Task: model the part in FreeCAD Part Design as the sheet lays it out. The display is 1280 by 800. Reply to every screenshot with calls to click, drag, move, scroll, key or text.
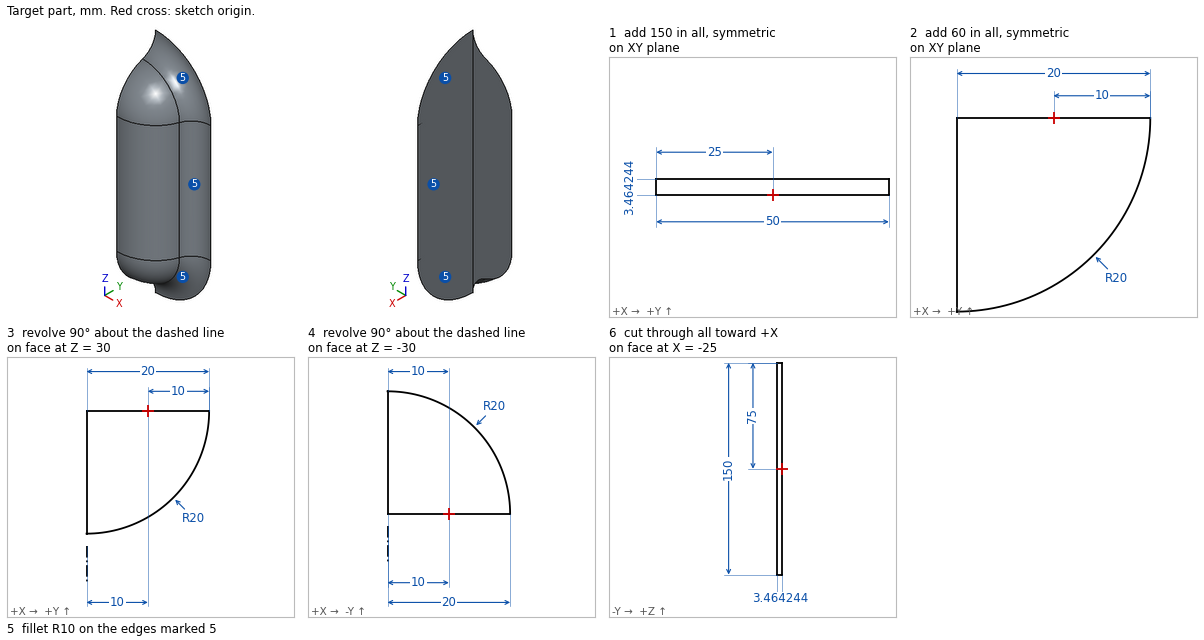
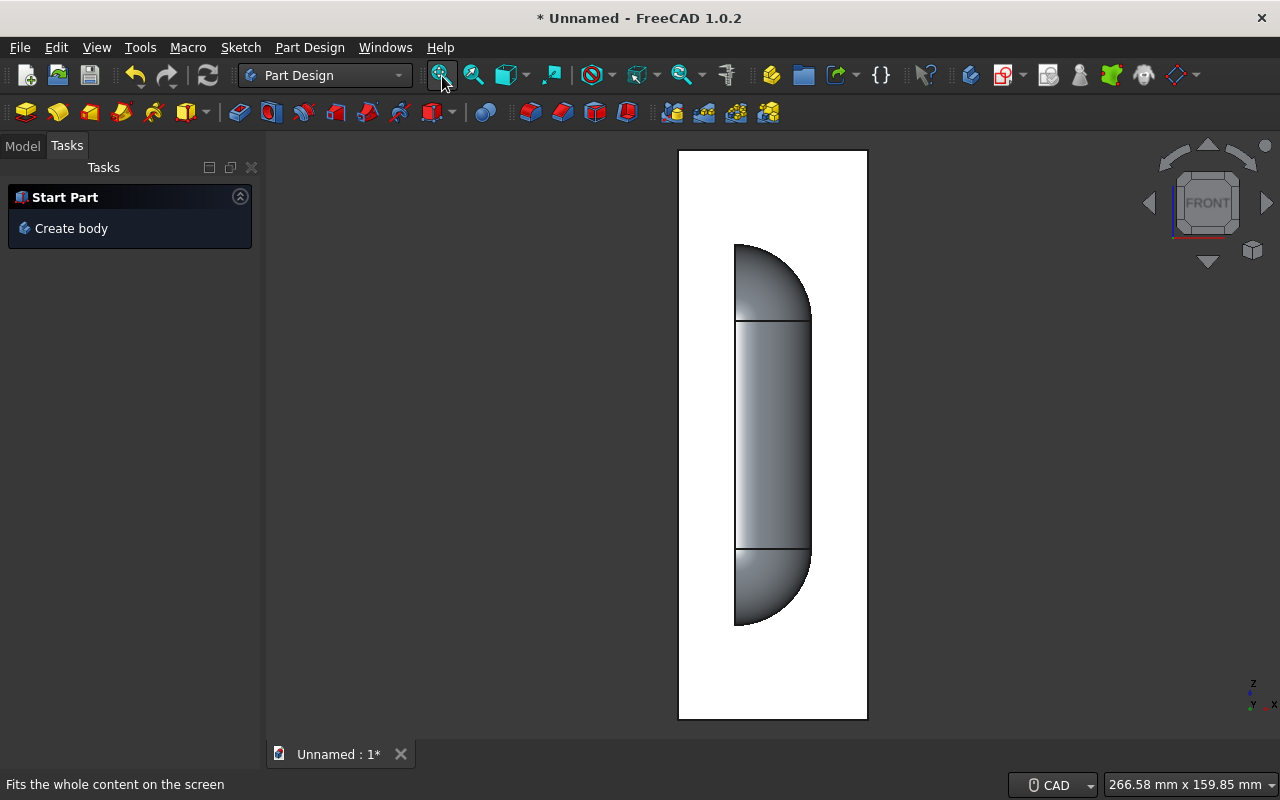
key(3)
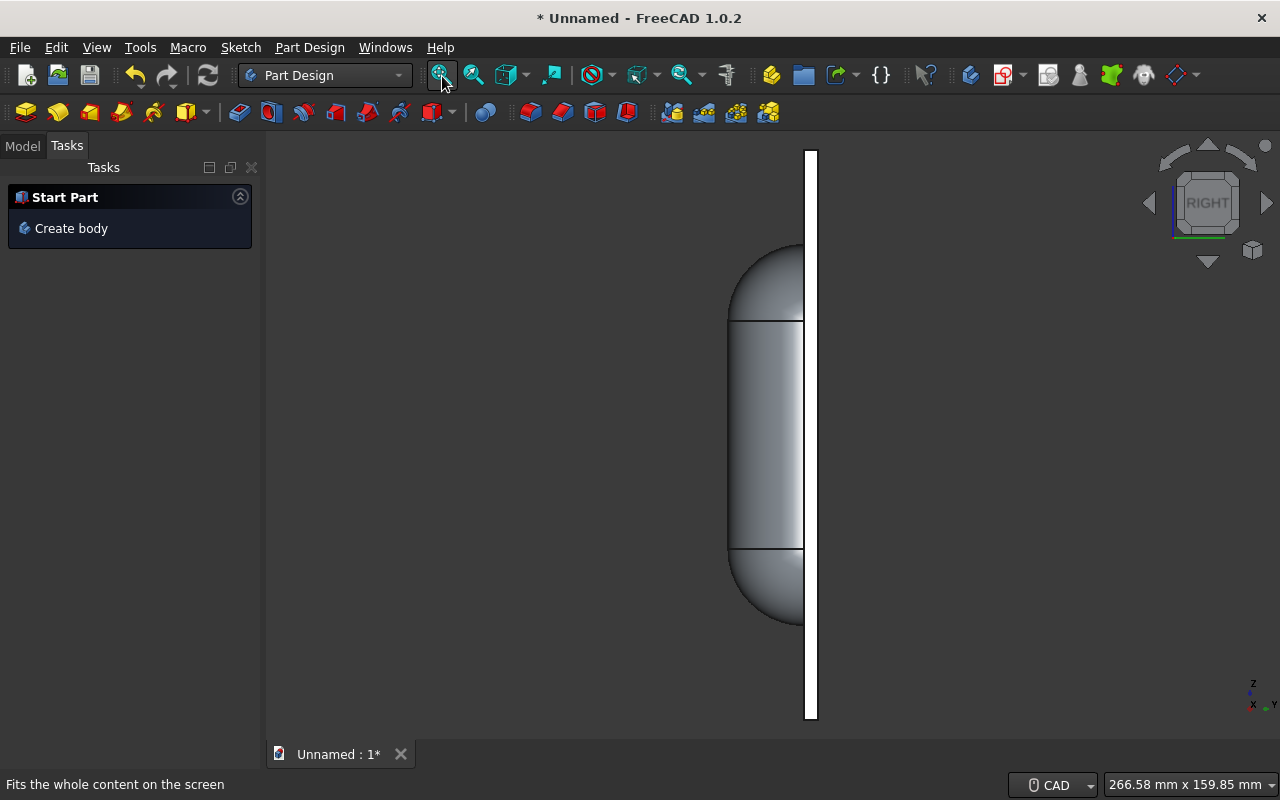
key(5)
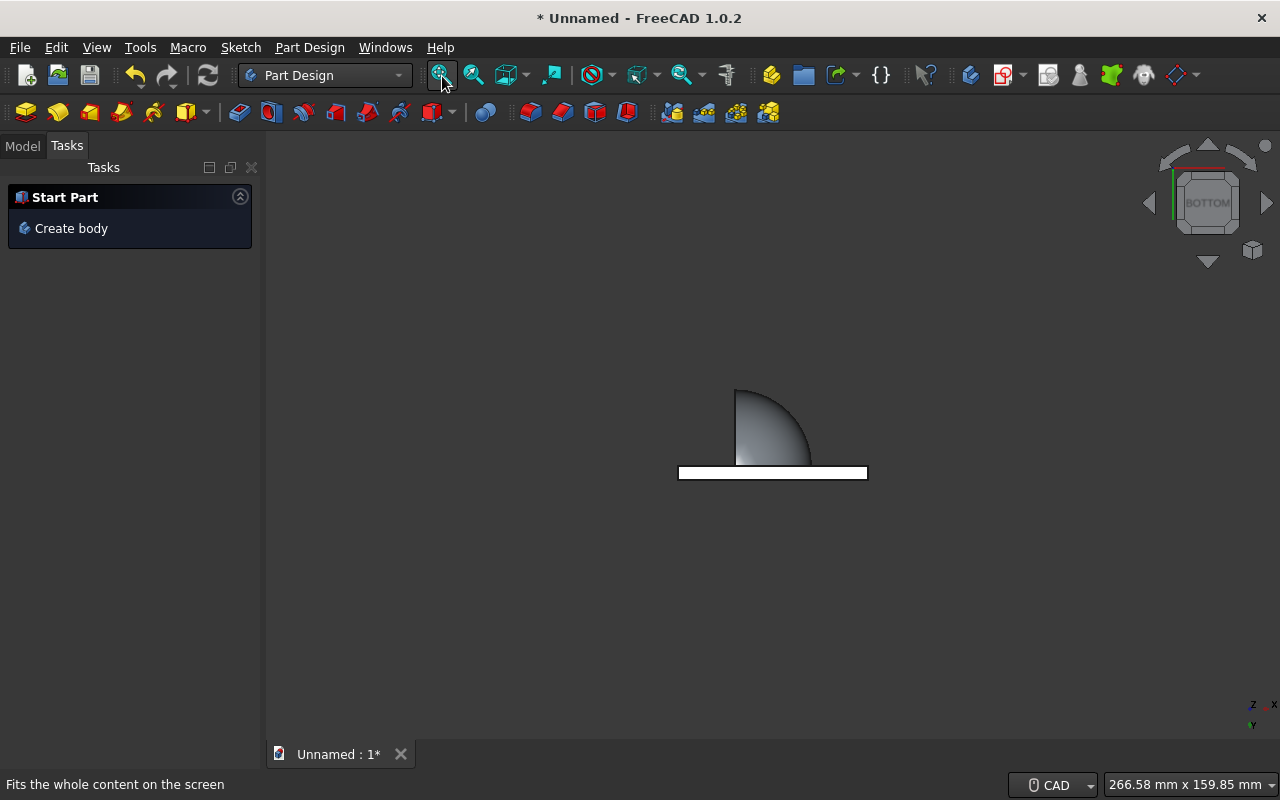
click(442, 76)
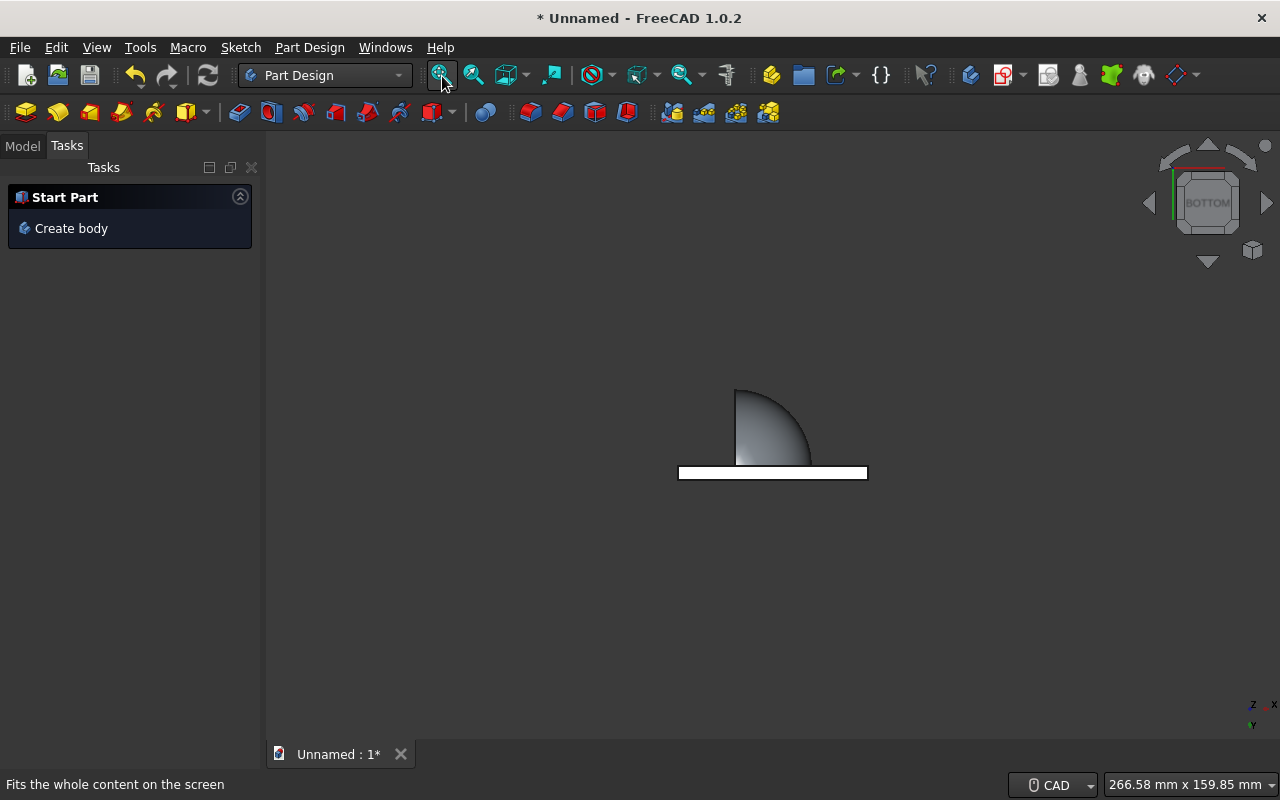
key(4)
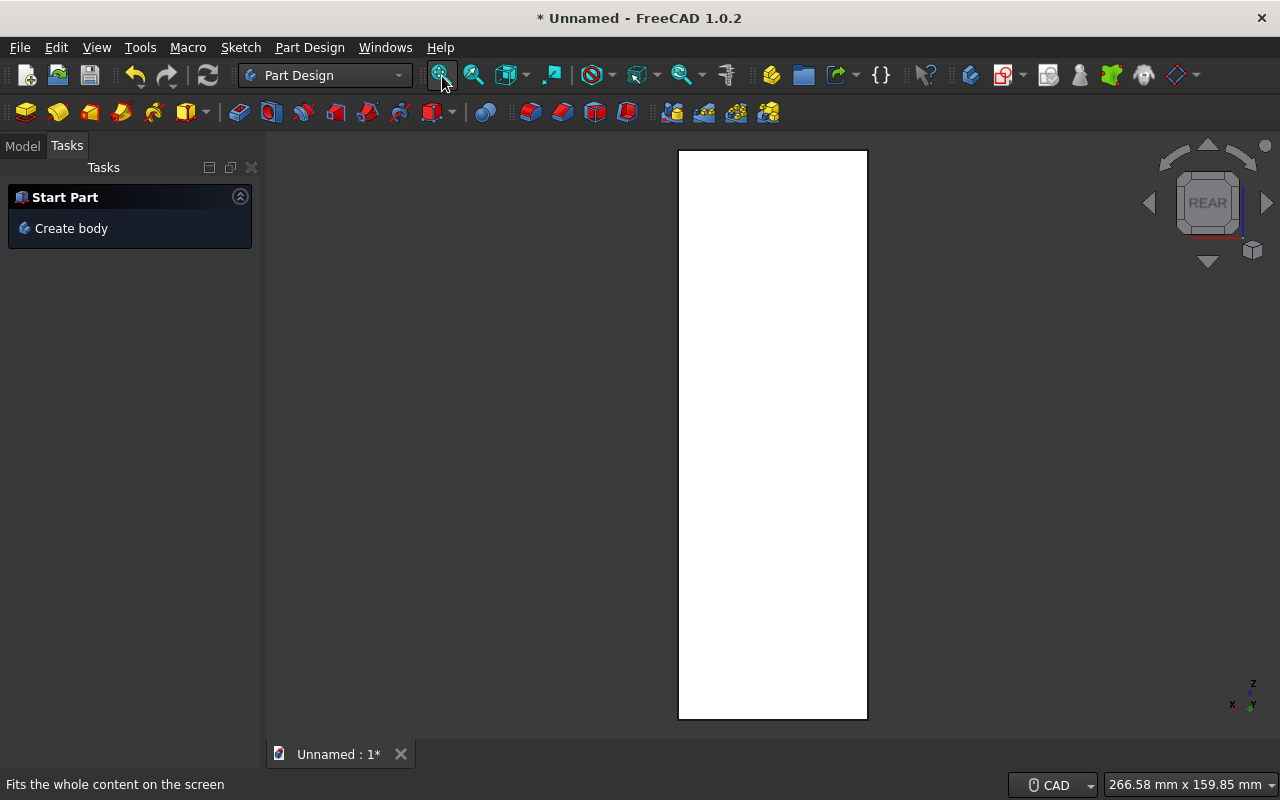
key(6)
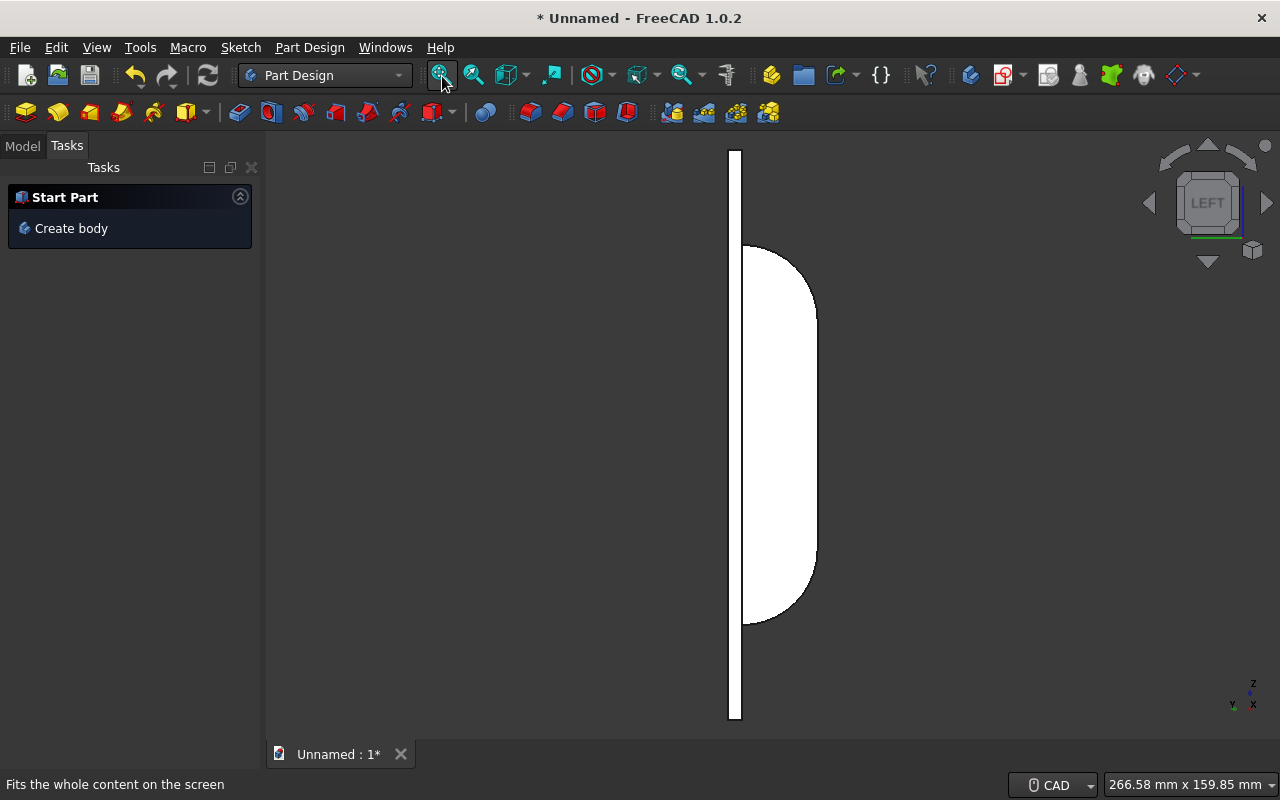
key(v)
key(3)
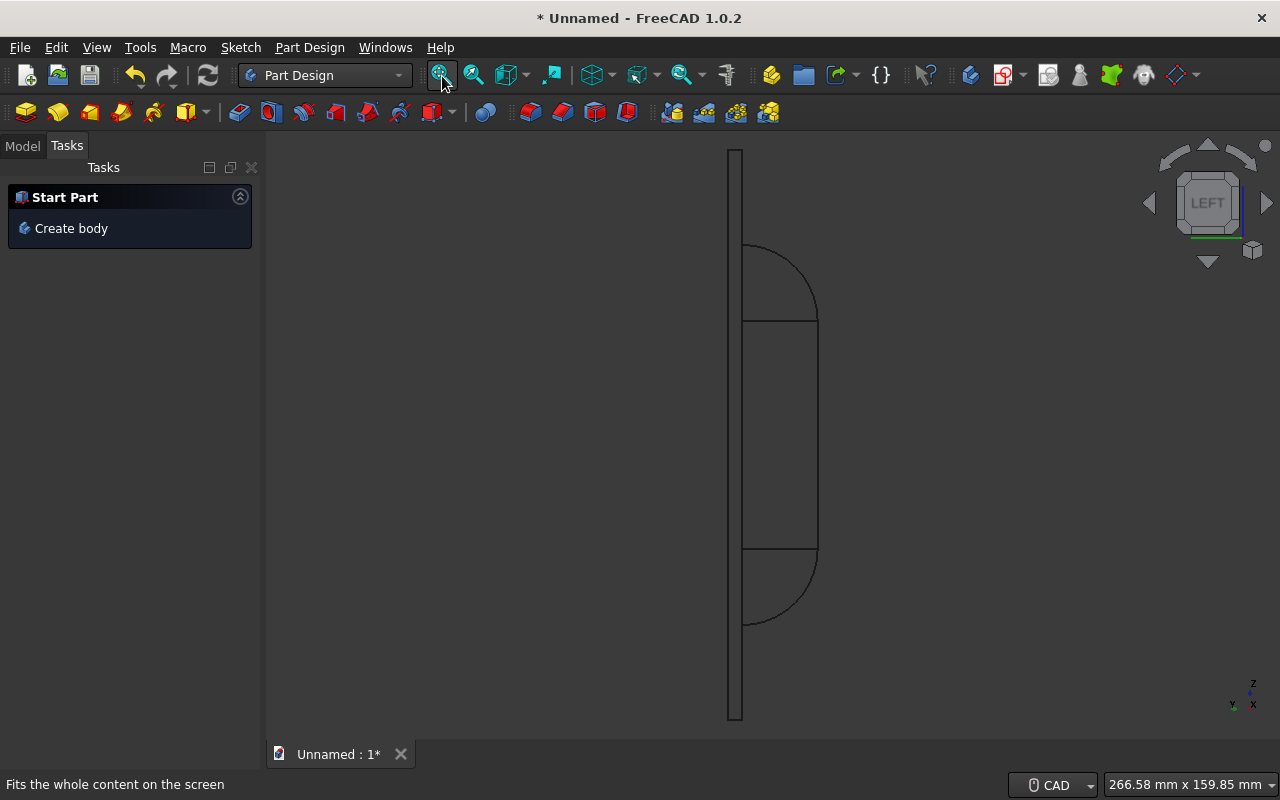
key(0)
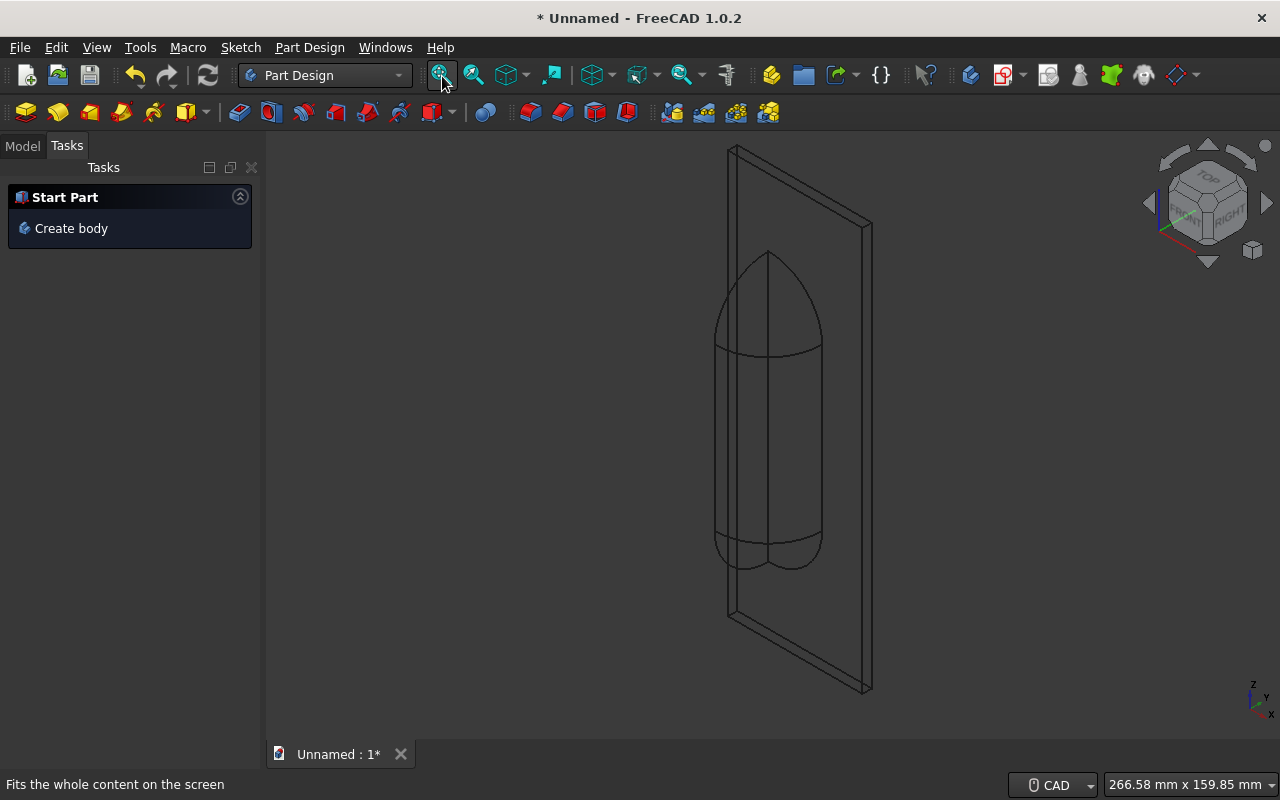
click(822, 437)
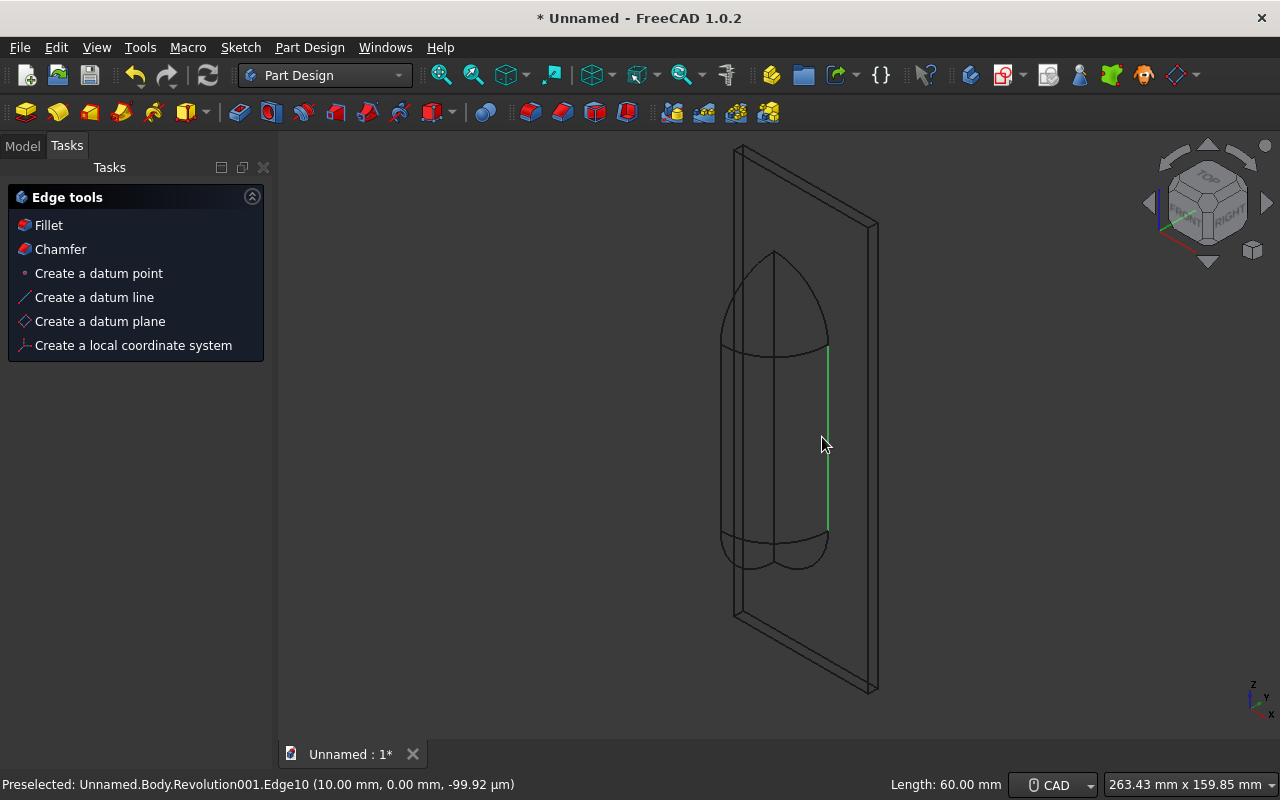
click(812, 291, ctrl)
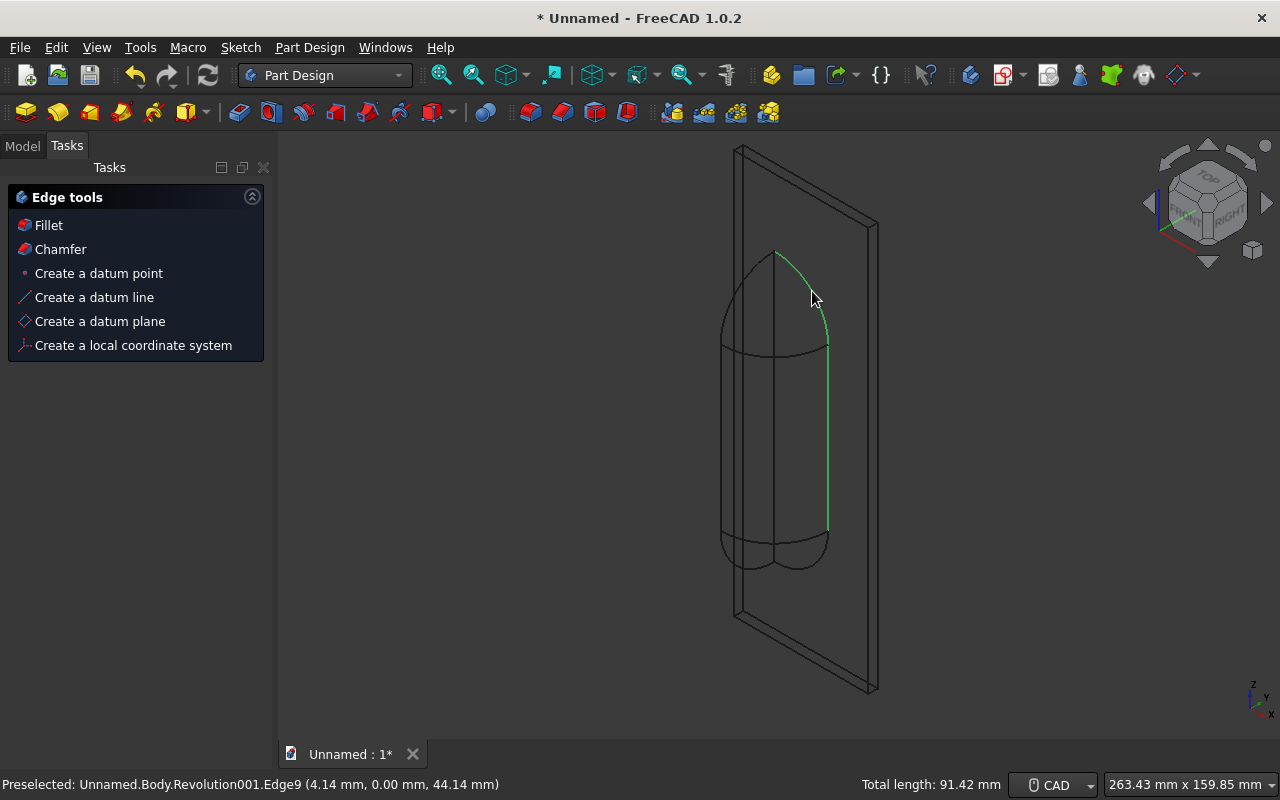
click(812, 565, ctrl)